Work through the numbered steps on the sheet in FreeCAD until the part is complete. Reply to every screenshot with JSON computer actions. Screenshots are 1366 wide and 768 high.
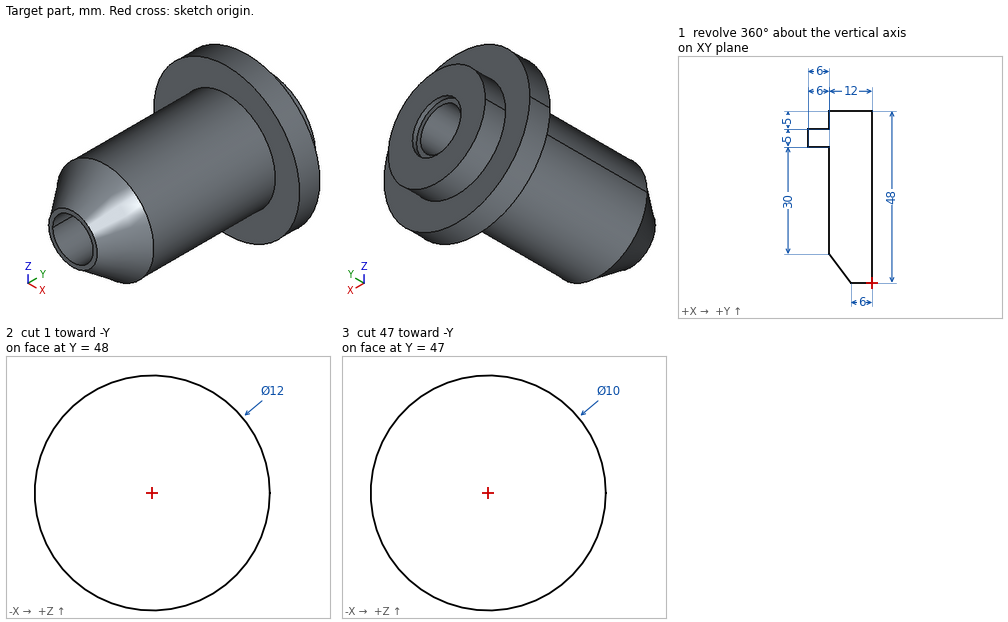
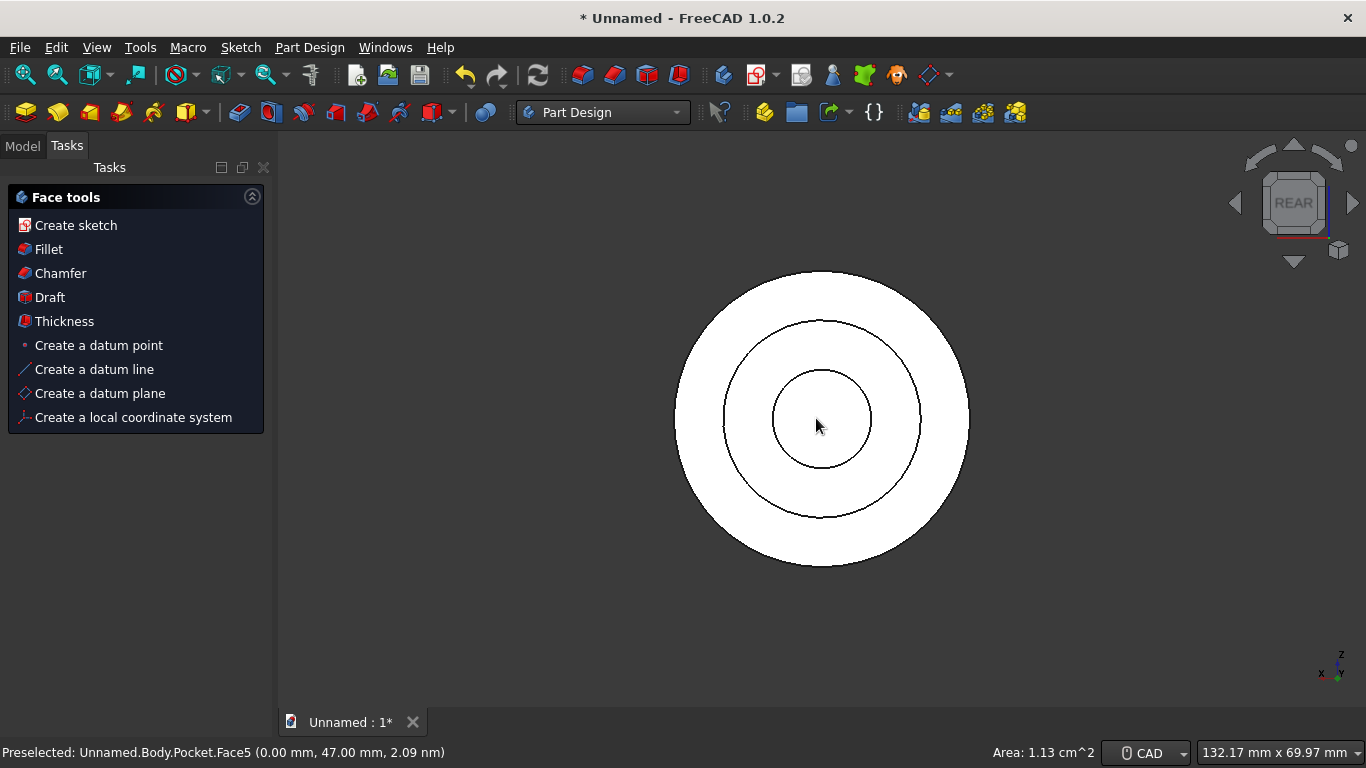
{"action": "left_click", "coordinate": [756, 76]}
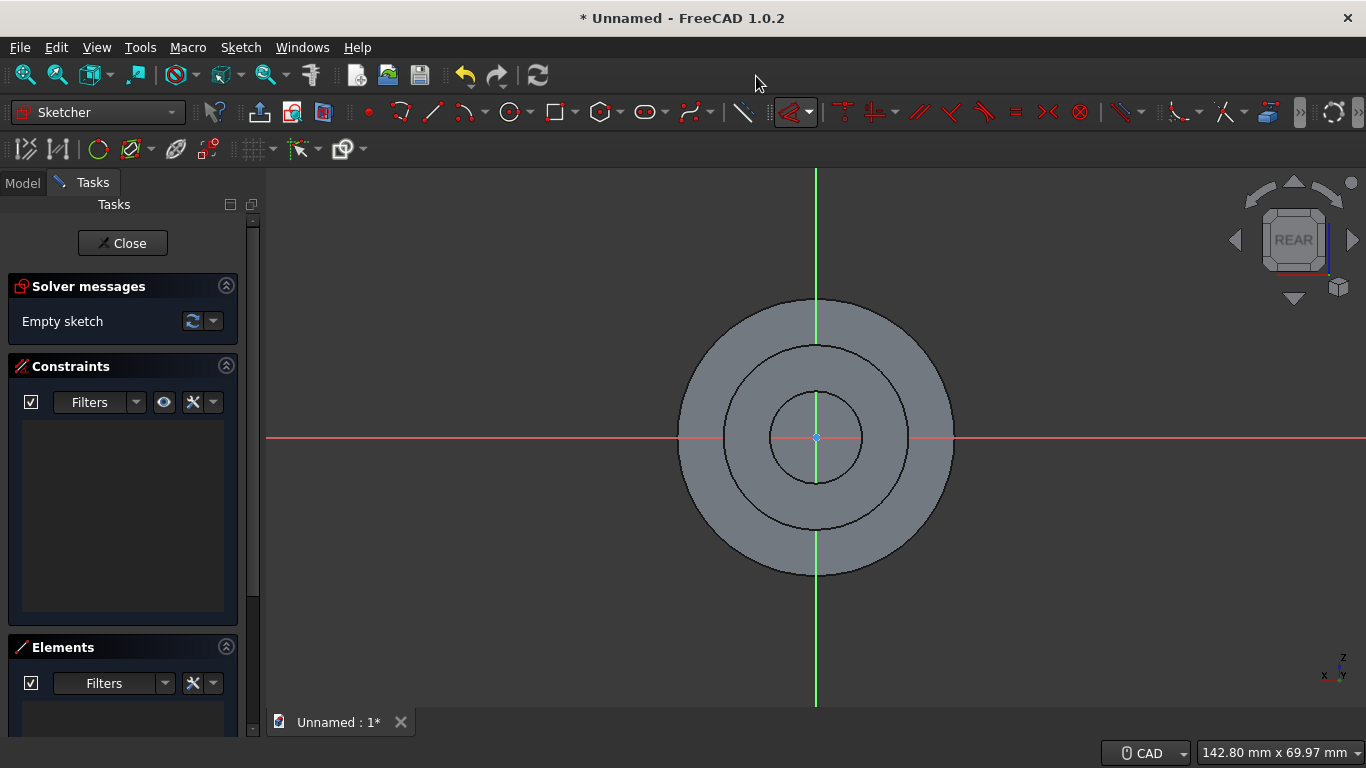
{"action": "scroll", "coordinate": [838, 438], "scroll_direction": "up", "scroll_amount": 7}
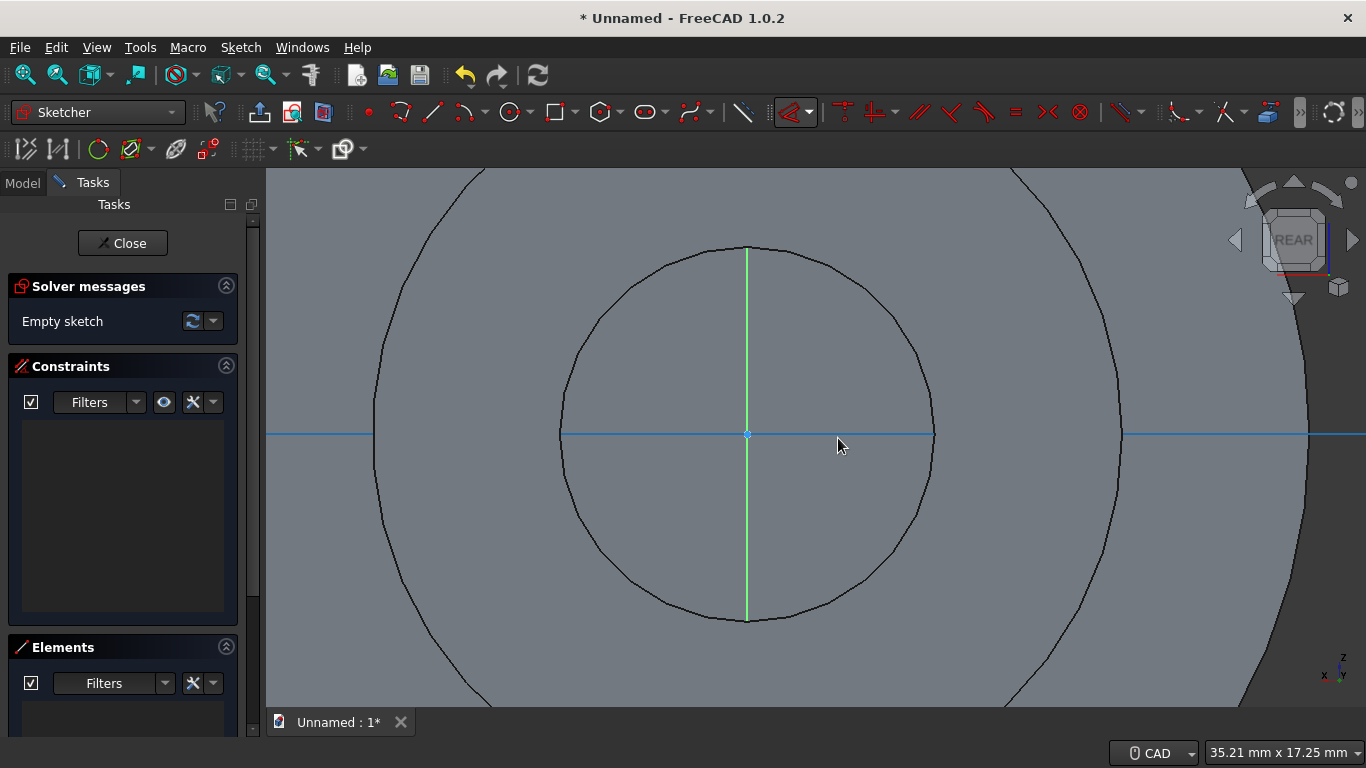
{"action": "left_click", "coordinate": [510, 112]}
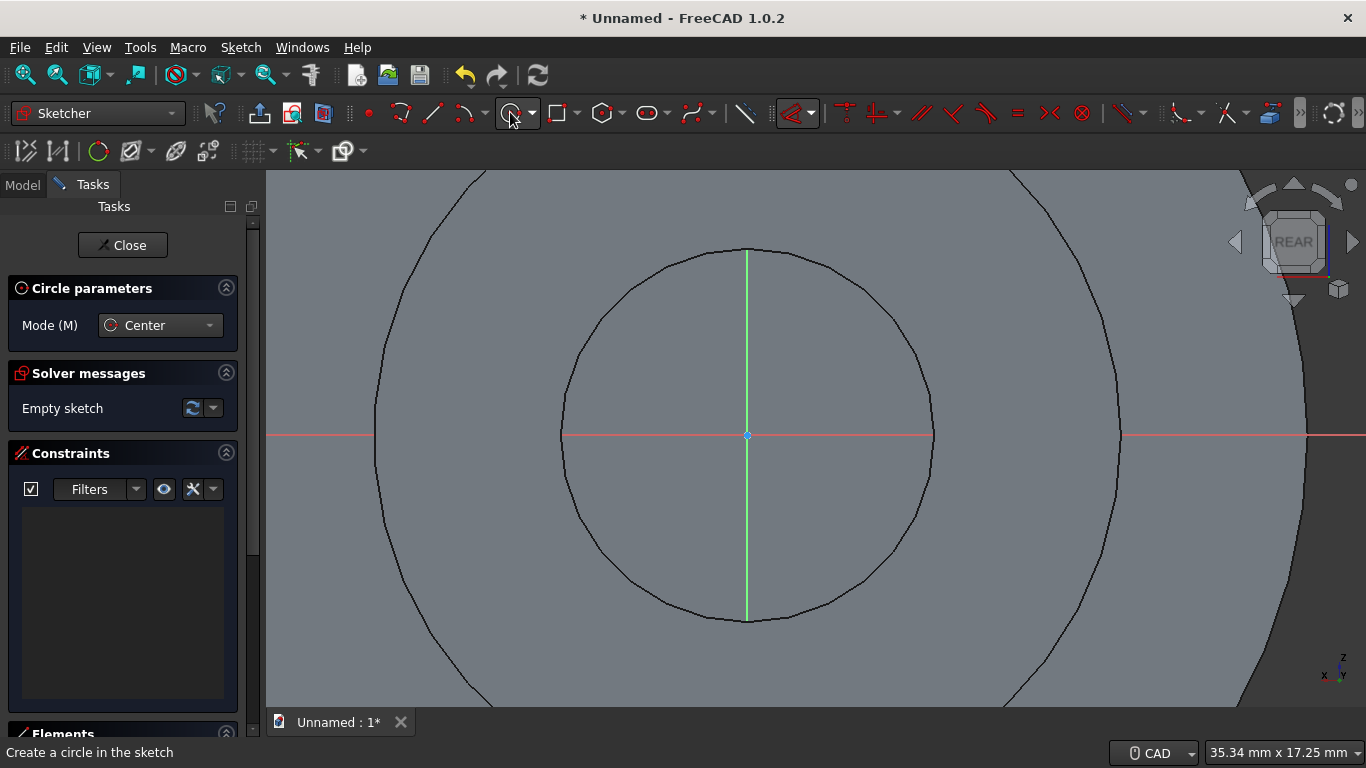
{"action": "left_click", "coordinate": [747, 435]}
{"action": "left_click", "coordinate": [857, 325]}
{"action": "key", "text": "Escape"}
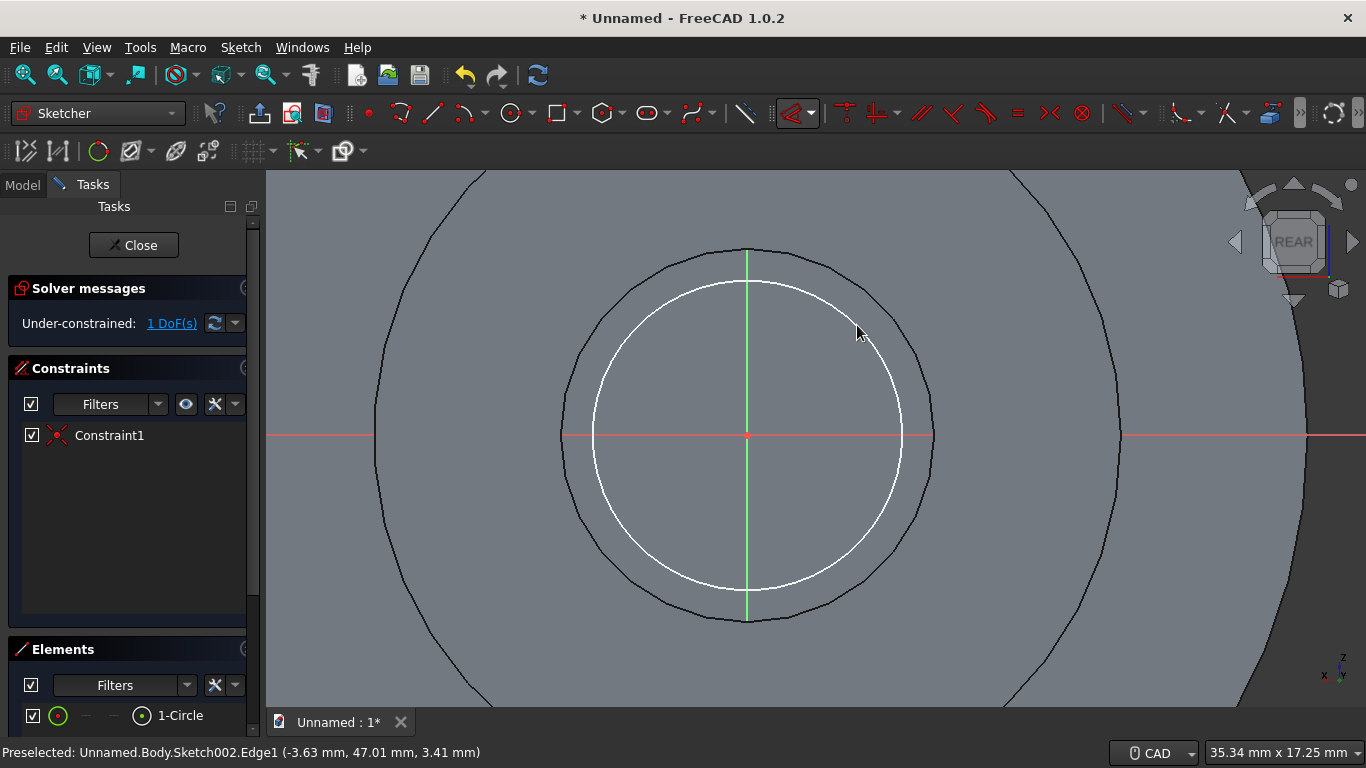
{"action": "left_click", "coordinate": [857, 326]}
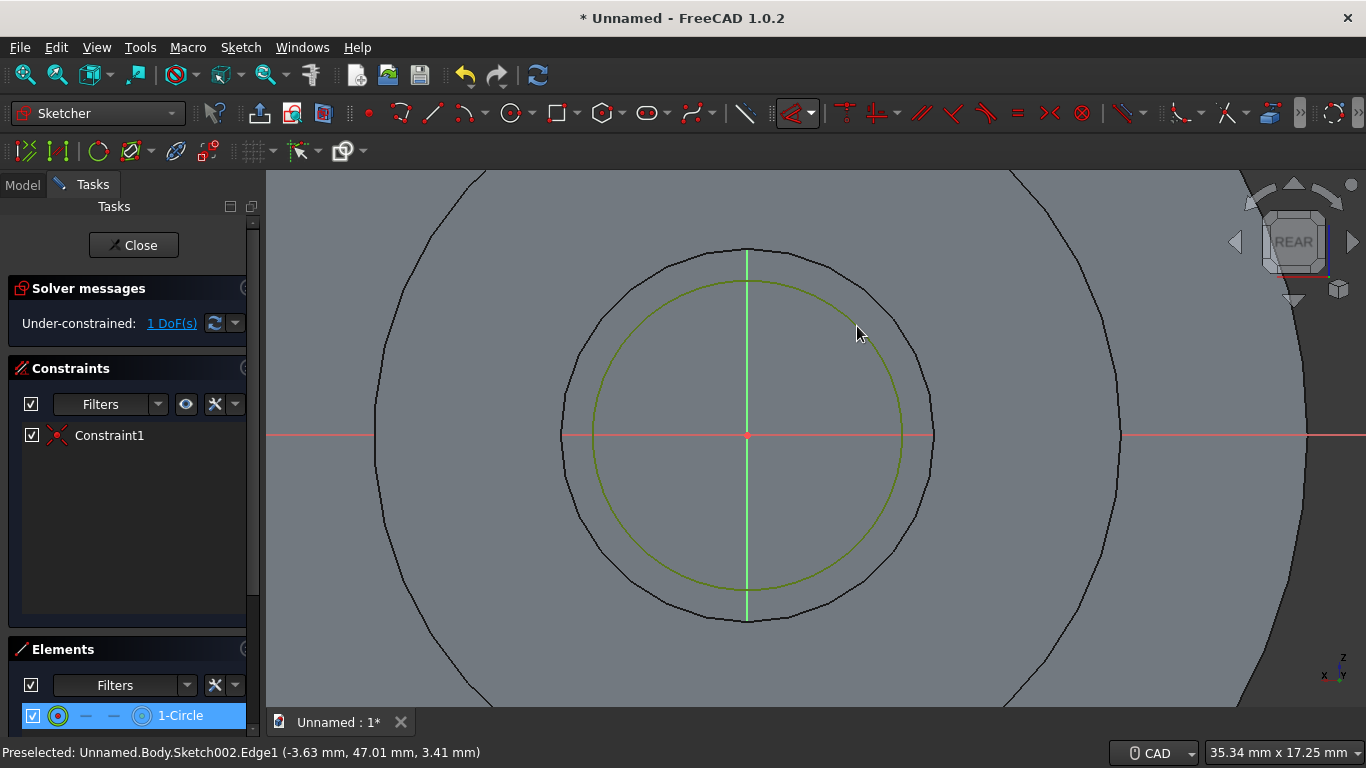
{"action": "left_click", "coordinate": [814, 114]}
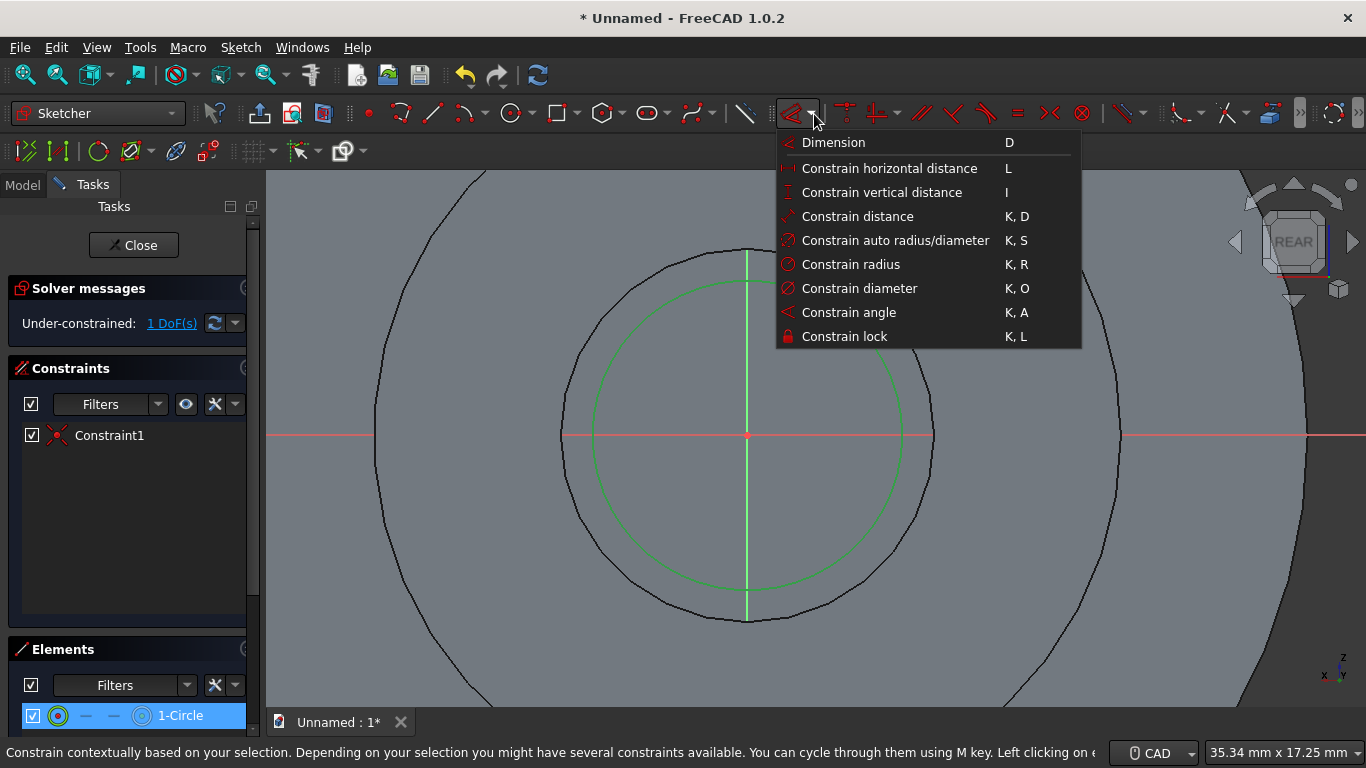
{"action": "left_click", "coordinate": [929, 288]}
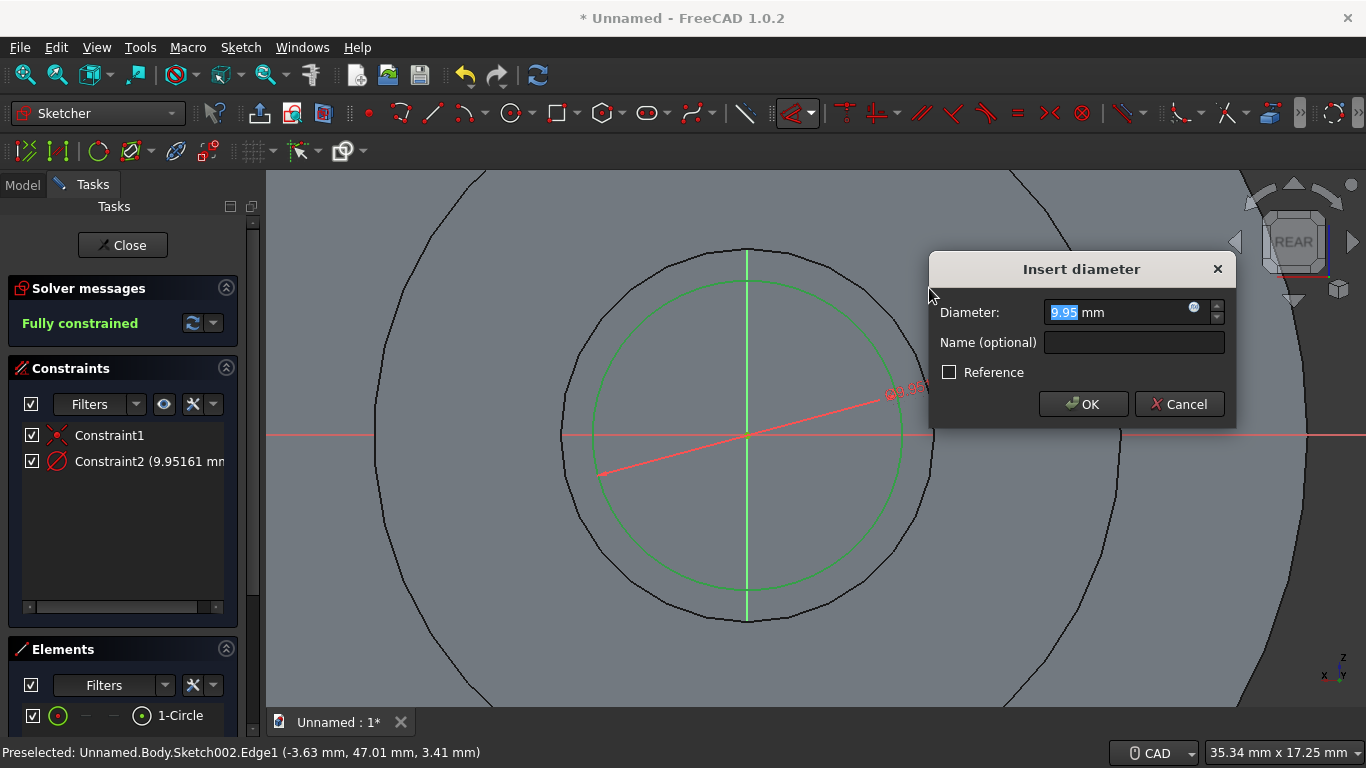
{"action": "type", "text": "10"}
{"action": "key", "text": "Return"}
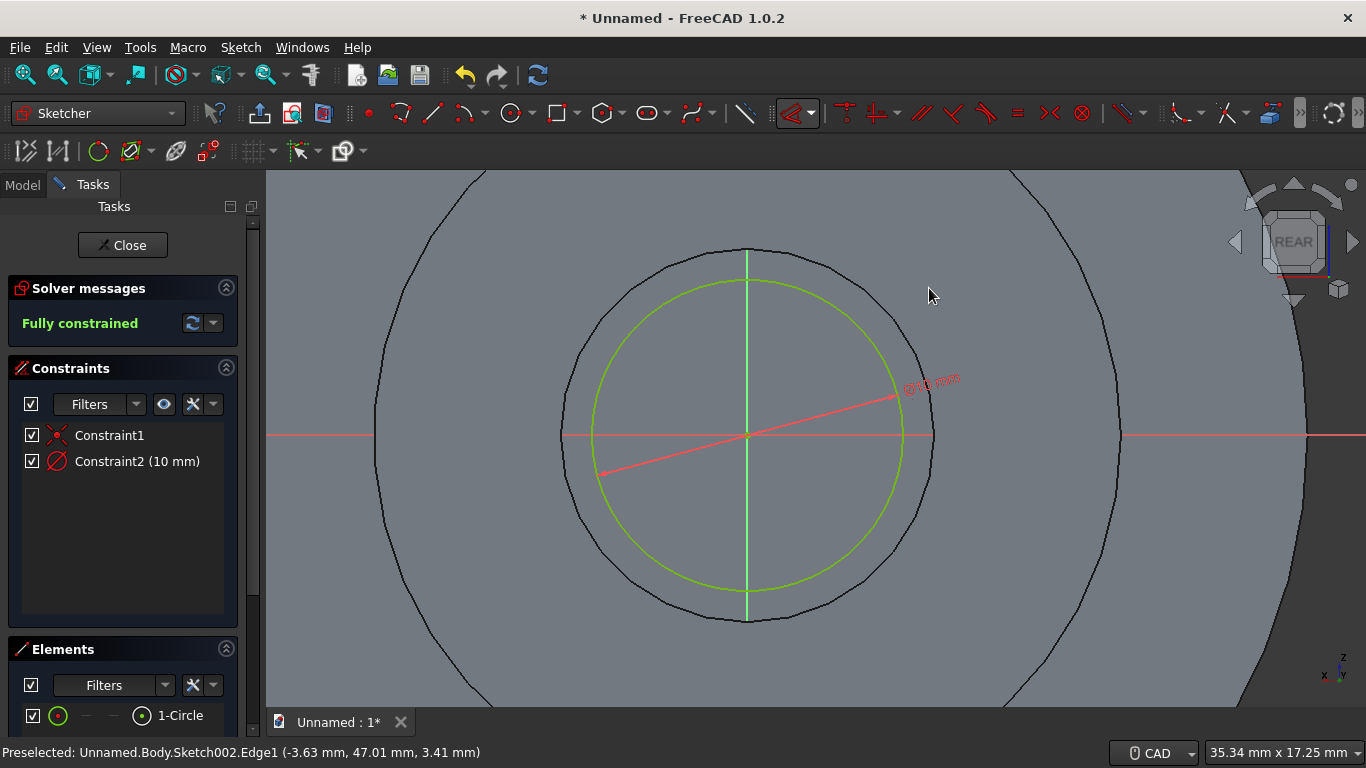
{"action": "left_click", "coordinate": [123, 245]}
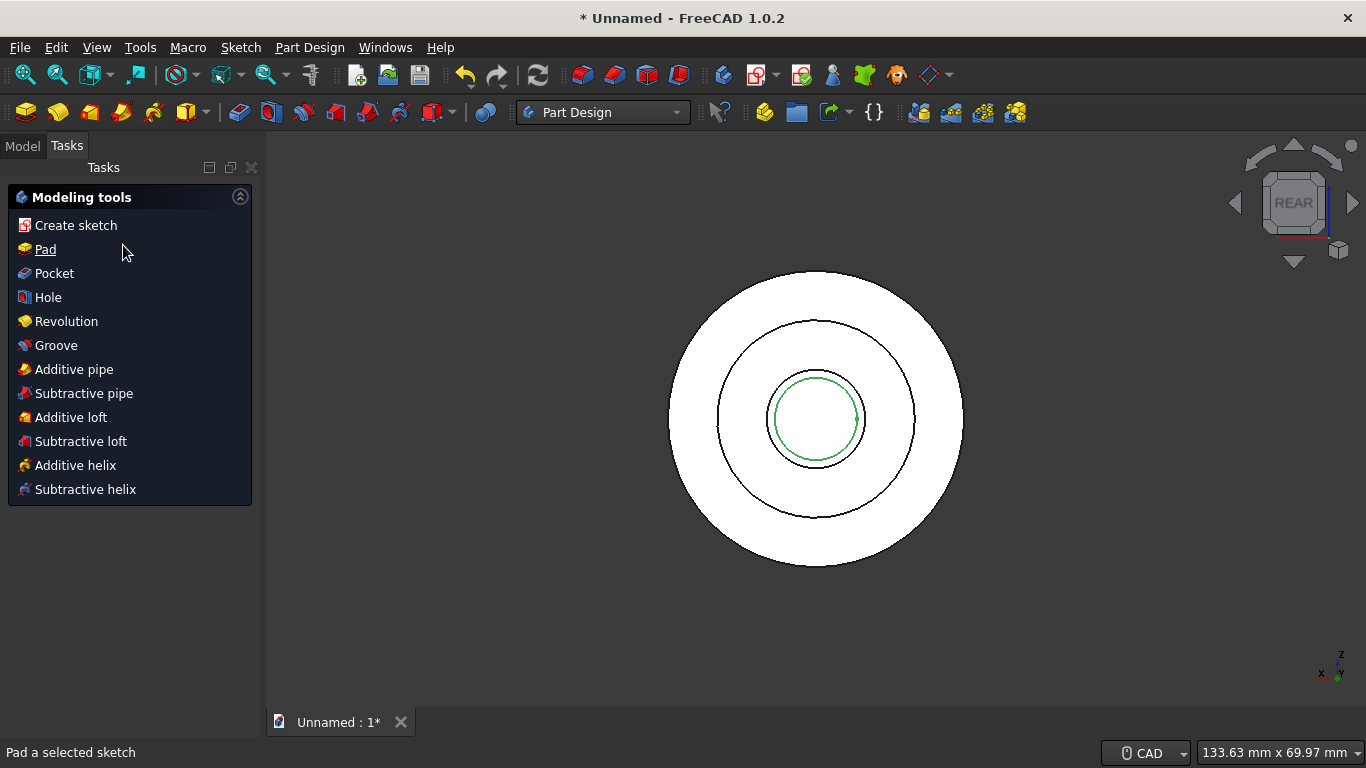
{"action": "left_click", "coordinate": [240, 112]}